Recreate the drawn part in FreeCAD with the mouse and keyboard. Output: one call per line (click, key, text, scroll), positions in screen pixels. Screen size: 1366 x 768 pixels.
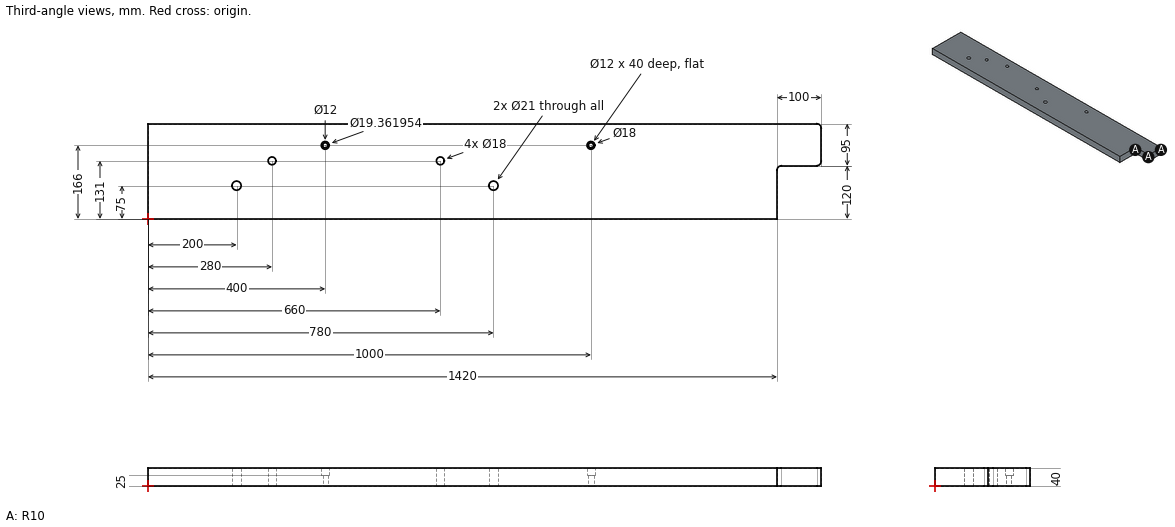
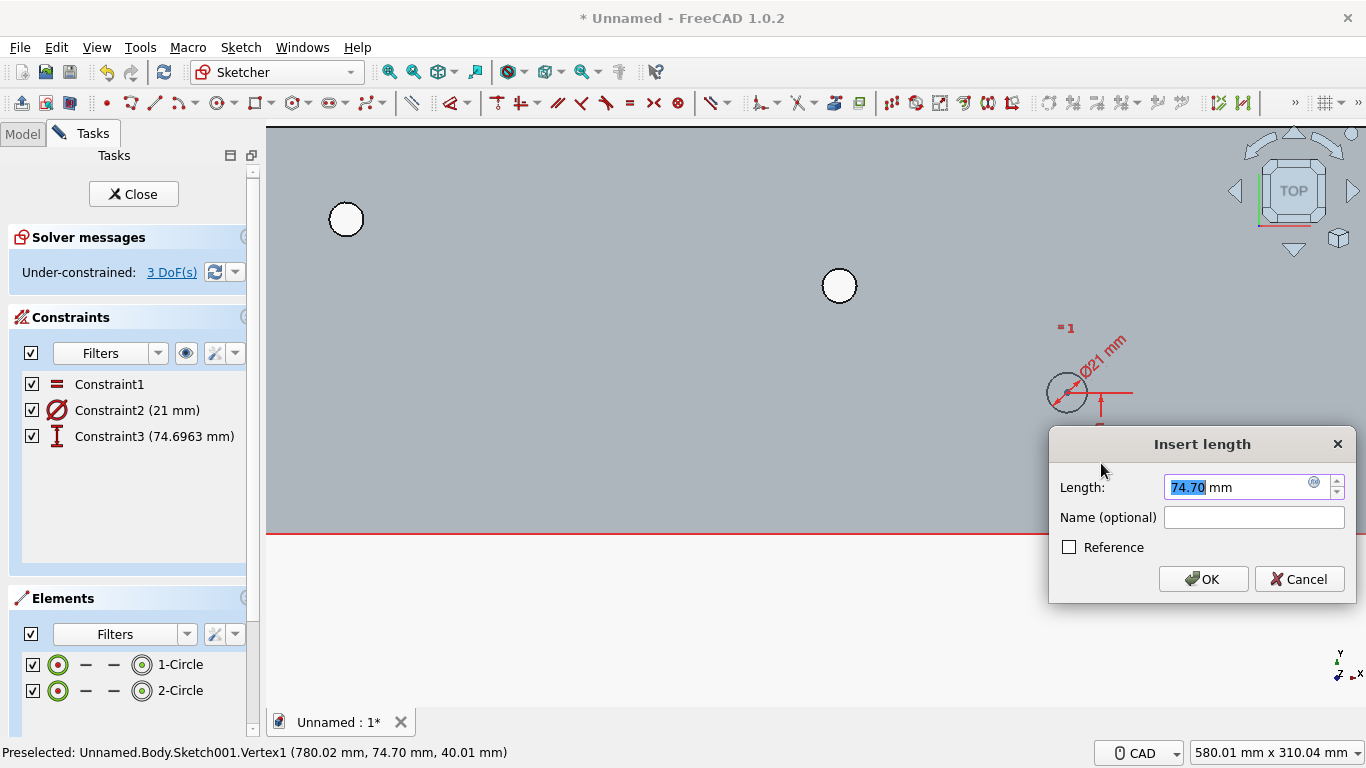
text(75)
key(Return)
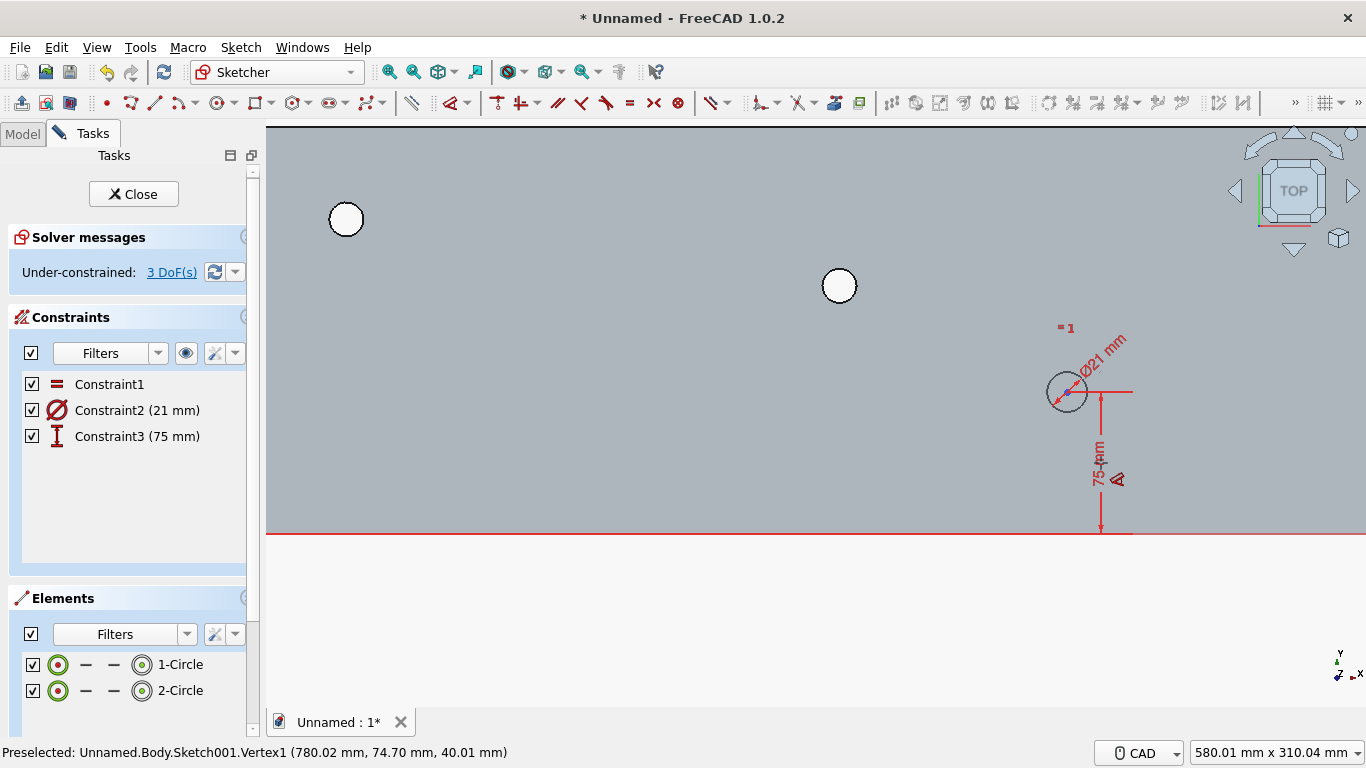
scroll(1082, 380, down, 4)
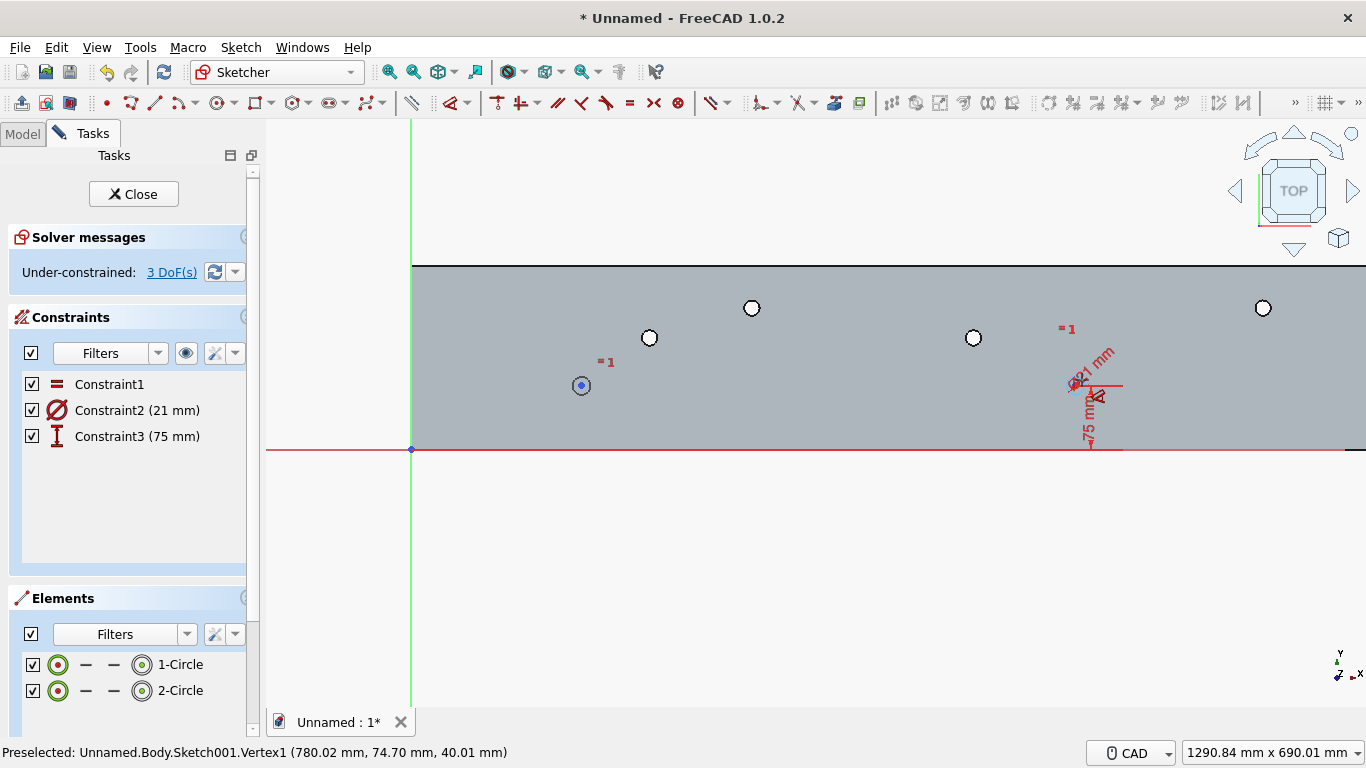
click(582, 386)
click(377, 418)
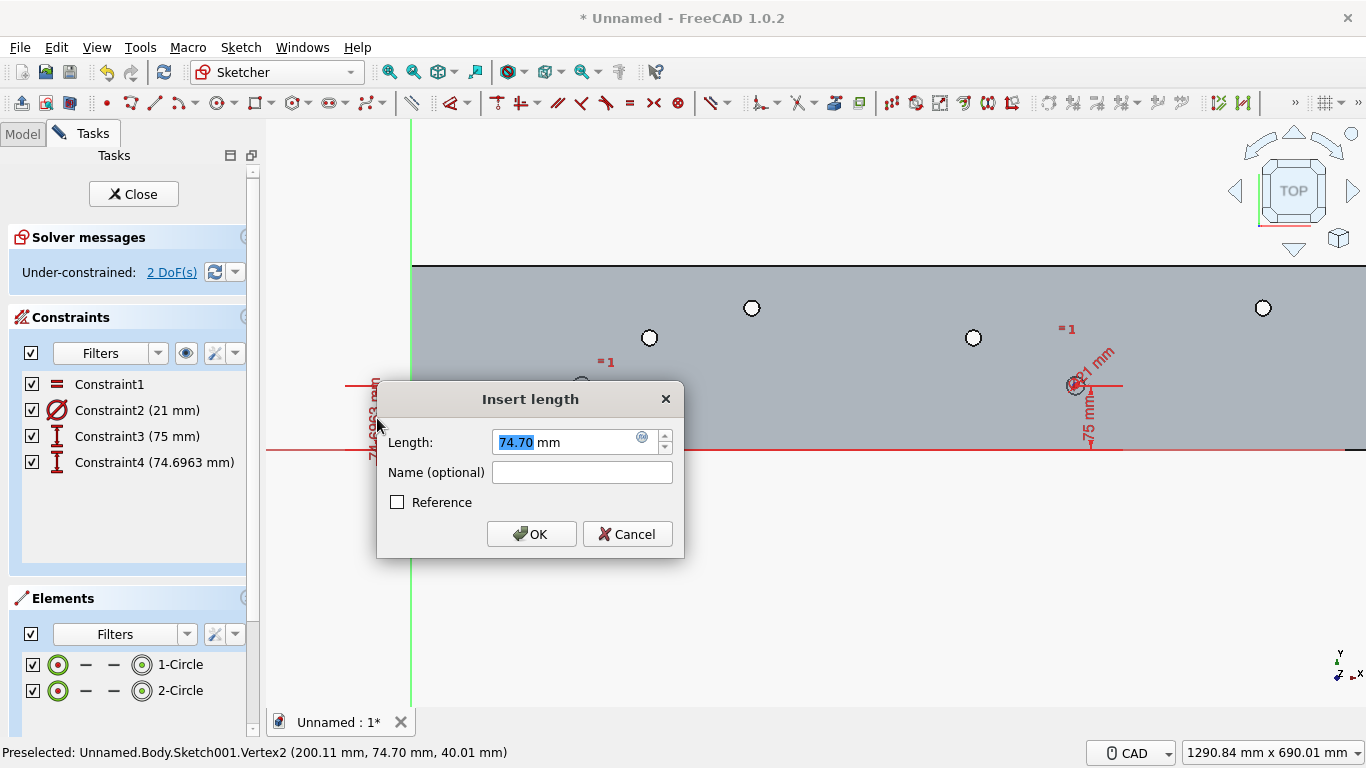
text(75)
key(Return)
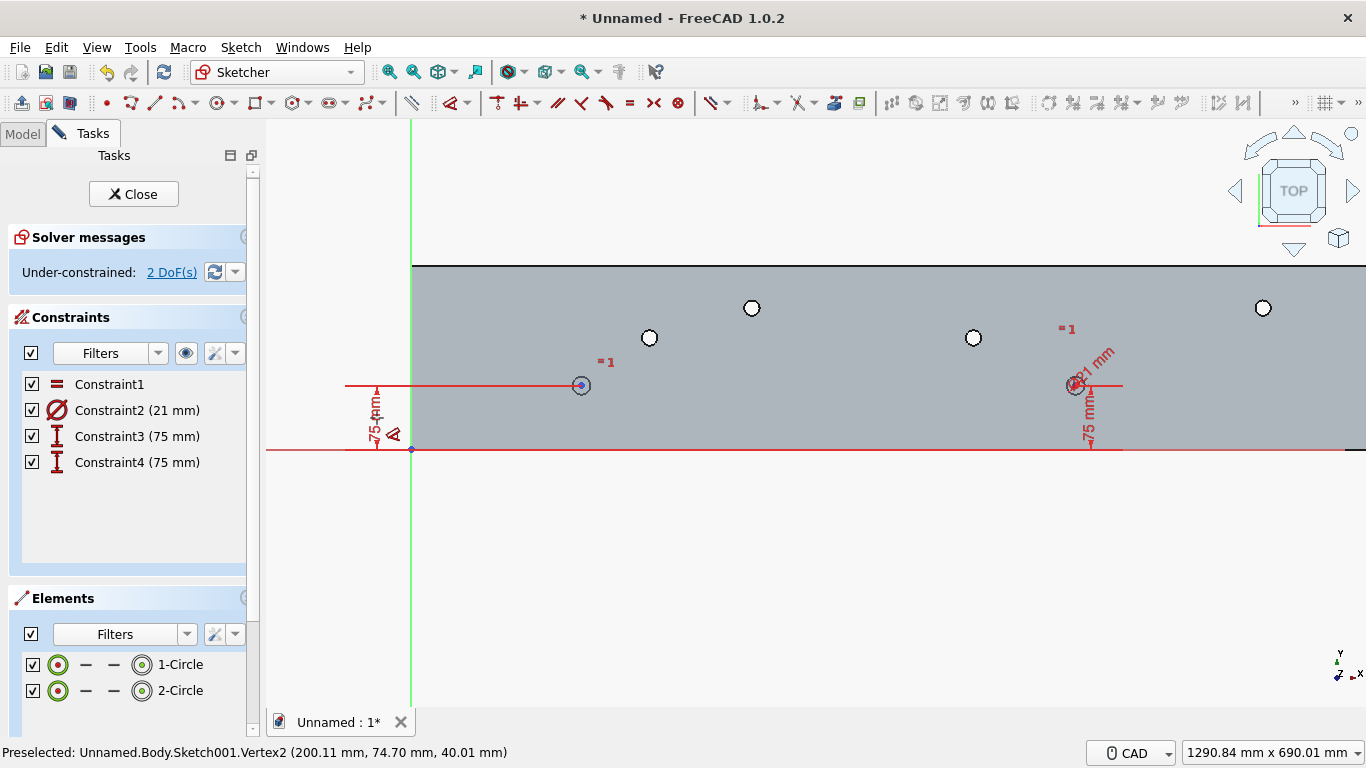
click(1076, 386)
click(743, 484)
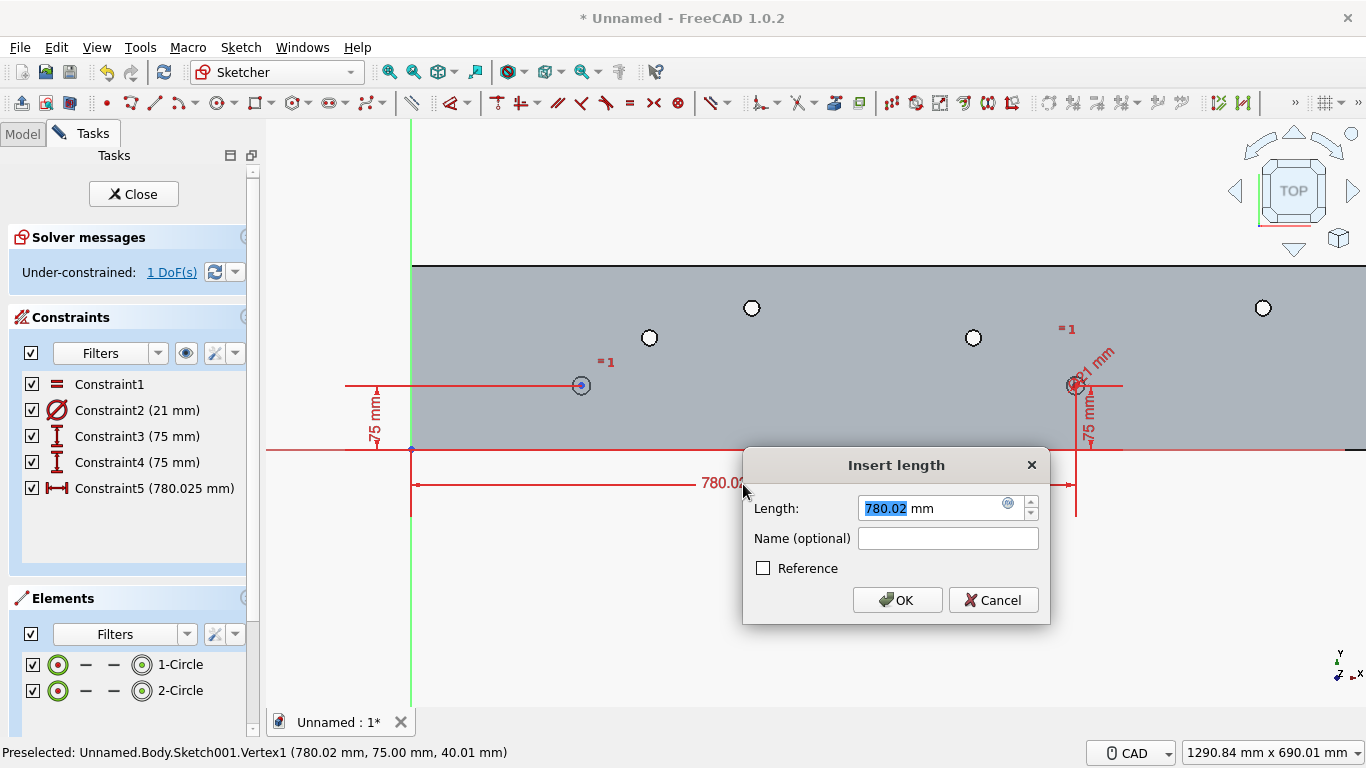
text(780)
key(Return)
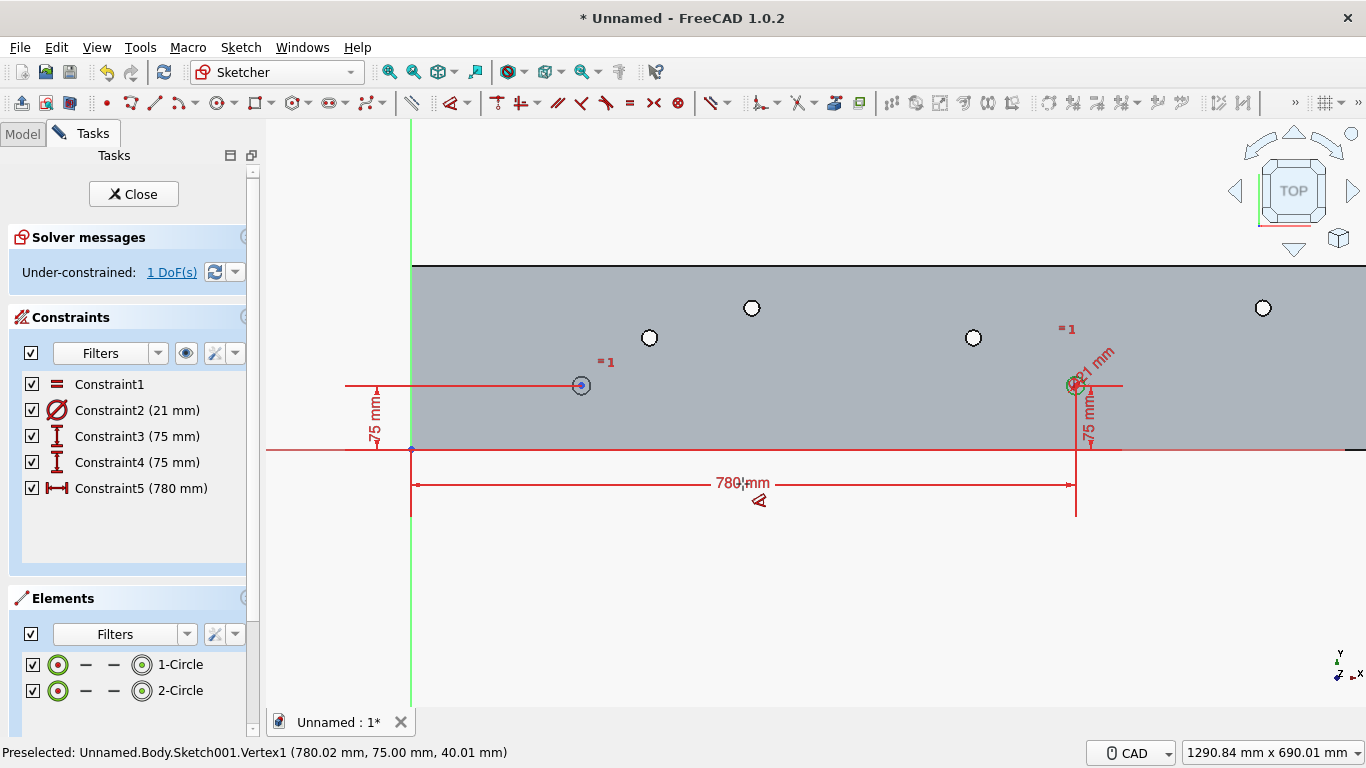
click(582, 386)
click(496, 484)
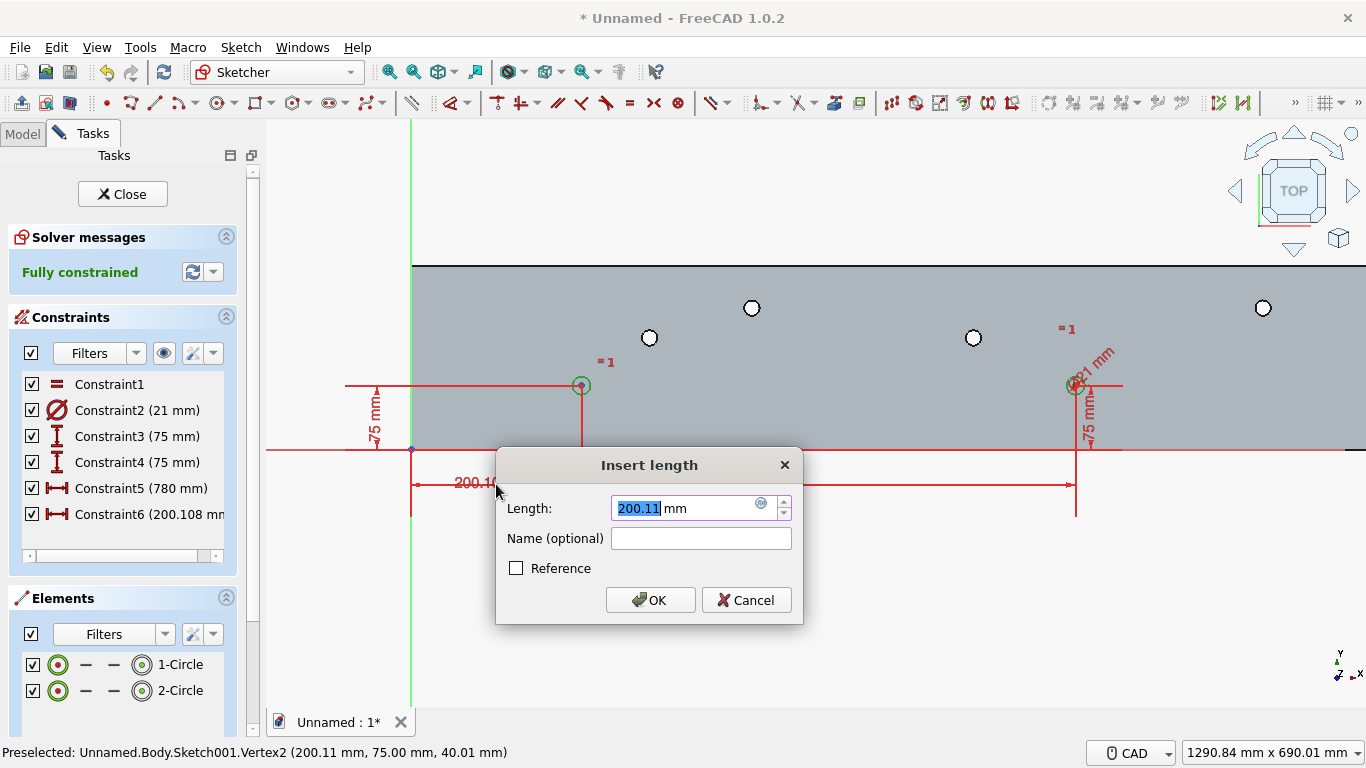
text(200)
key(Return)
key(Escape)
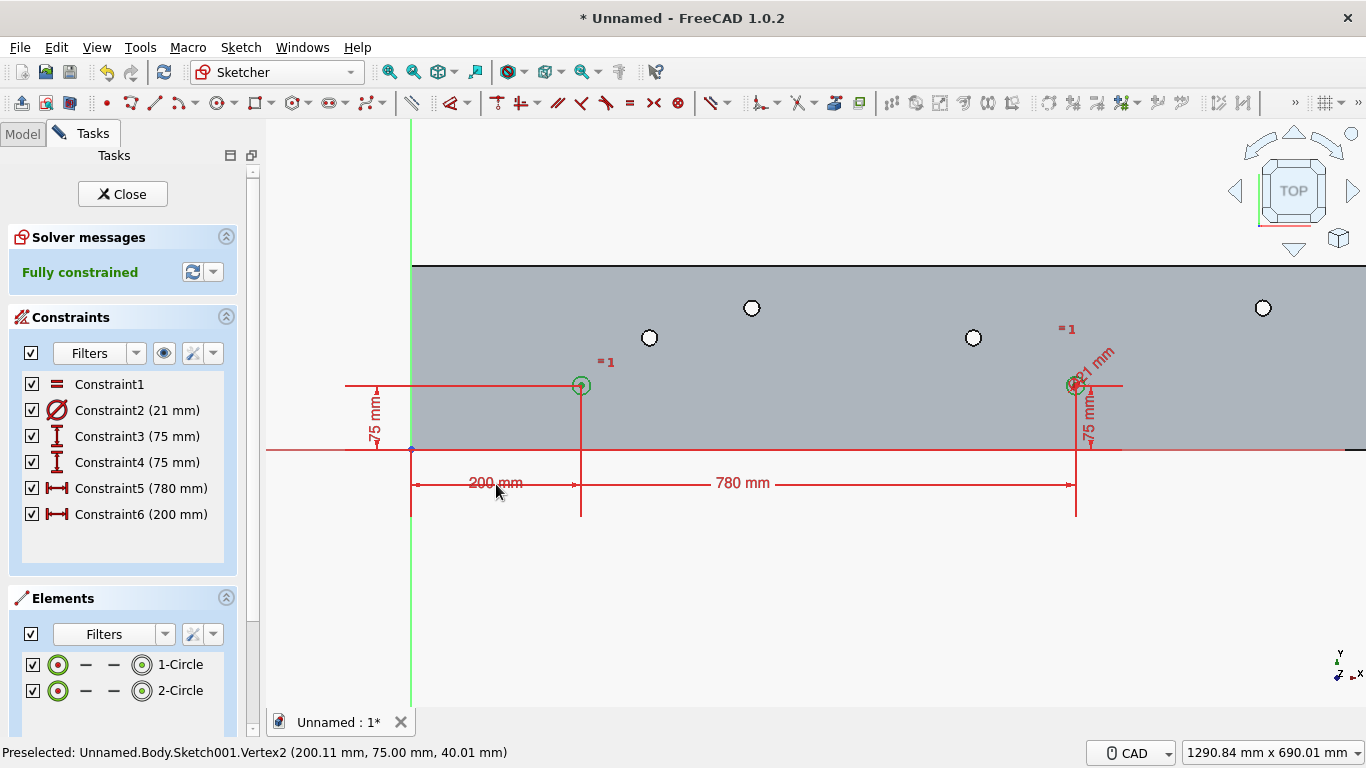
click(123, 194)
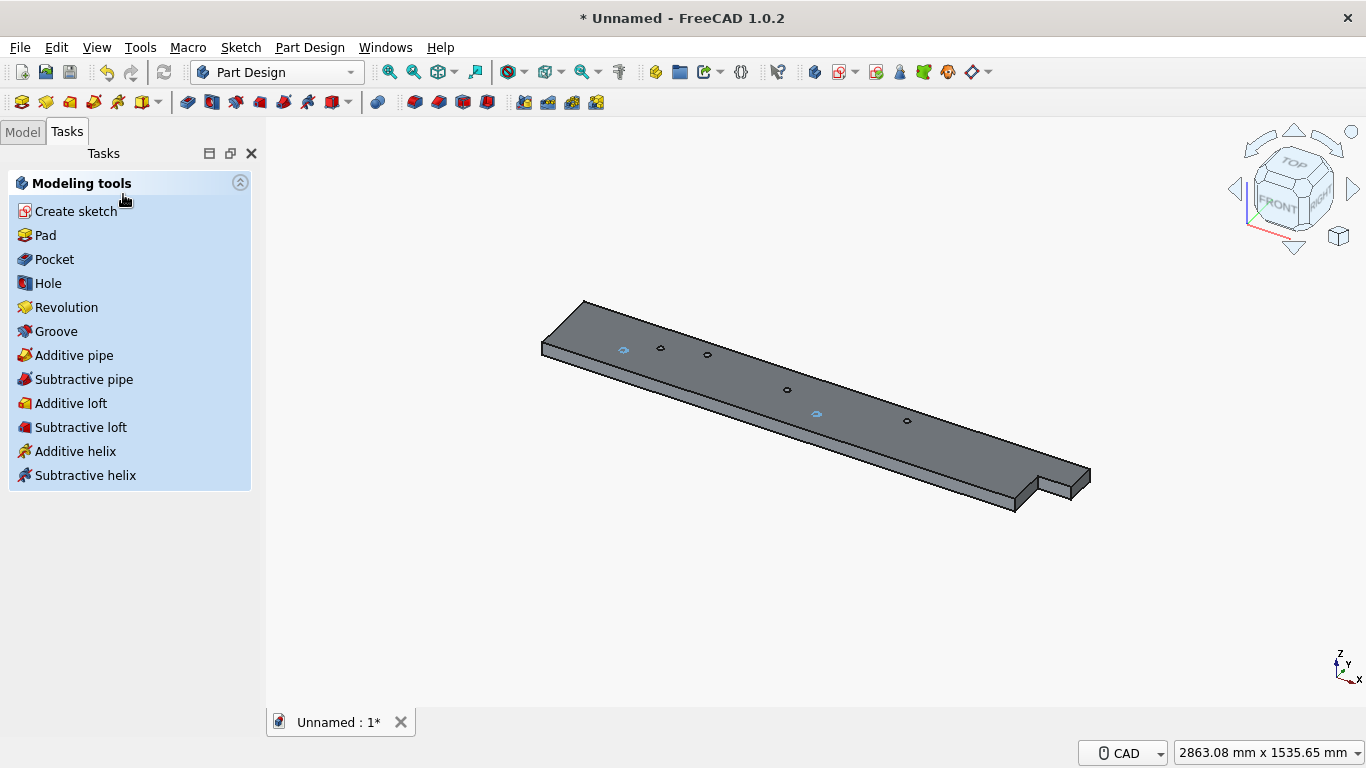
click(212, 102)